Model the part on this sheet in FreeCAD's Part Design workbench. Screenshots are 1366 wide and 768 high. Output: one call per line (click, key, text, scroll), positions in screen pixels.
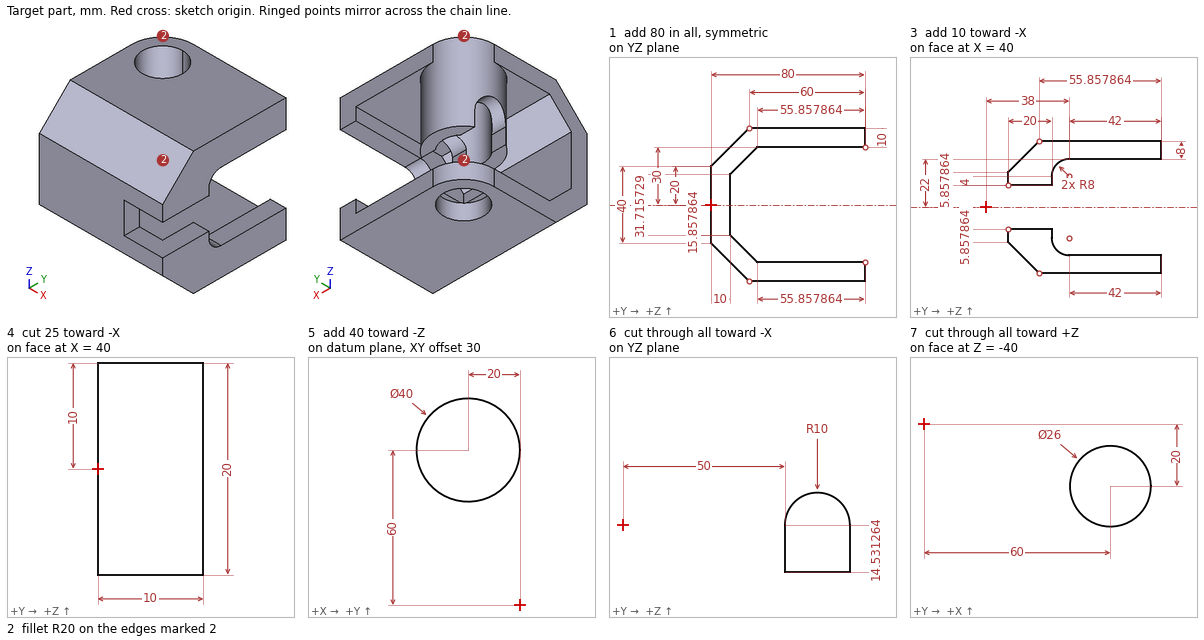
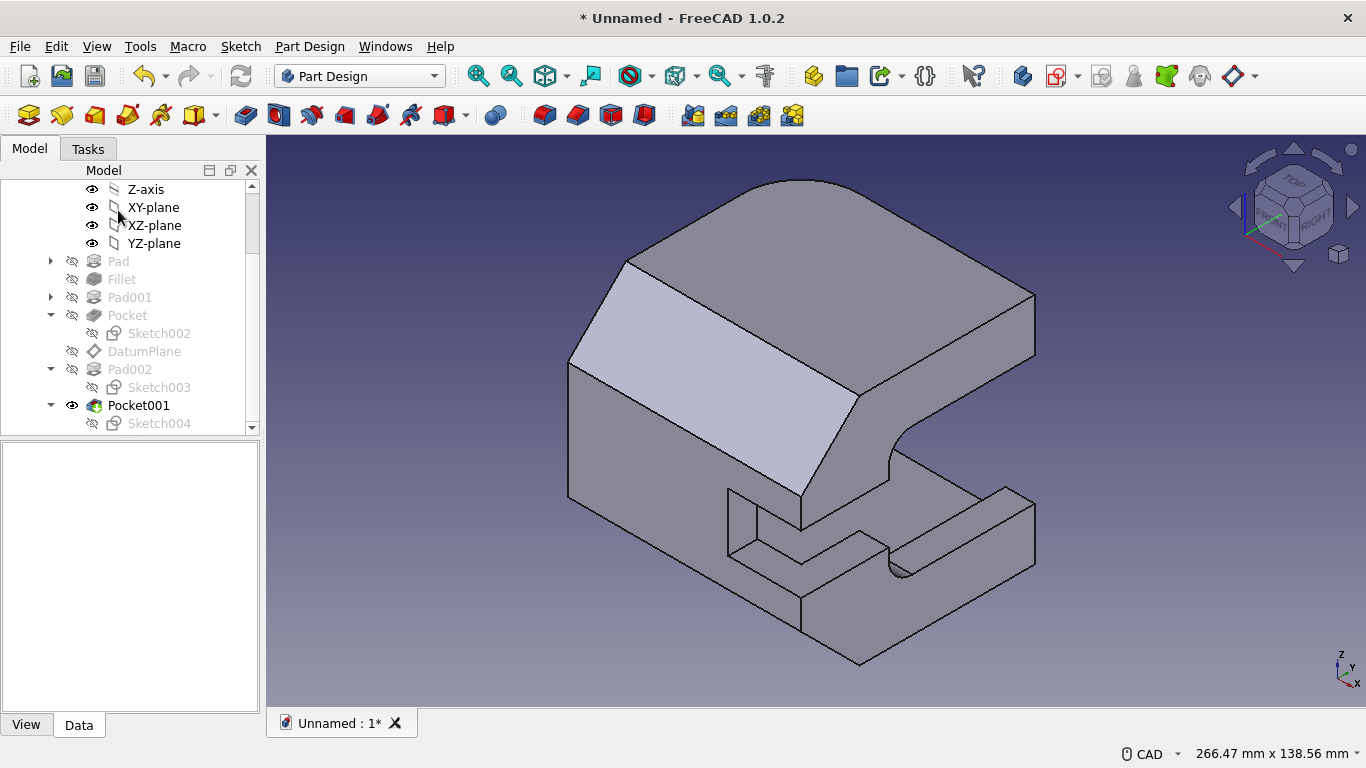
key(5)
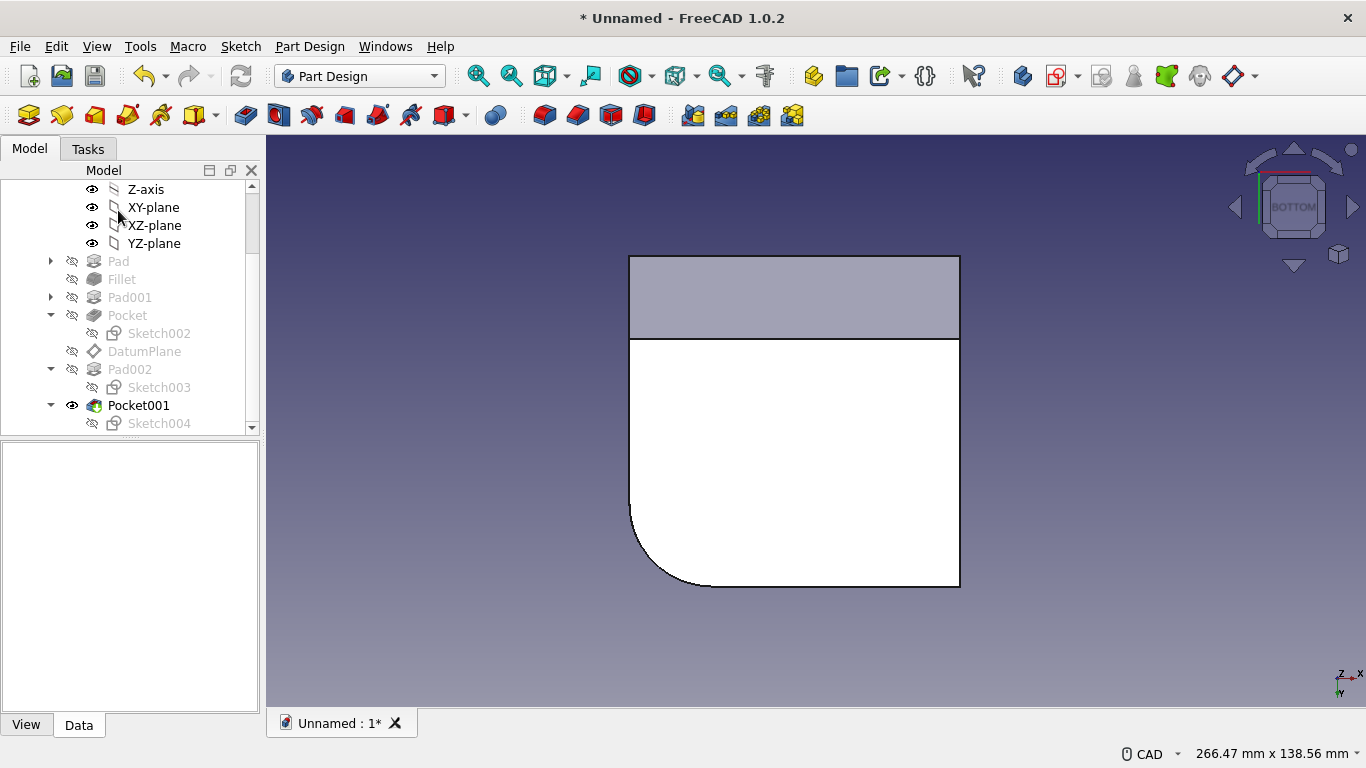
click(795, 462)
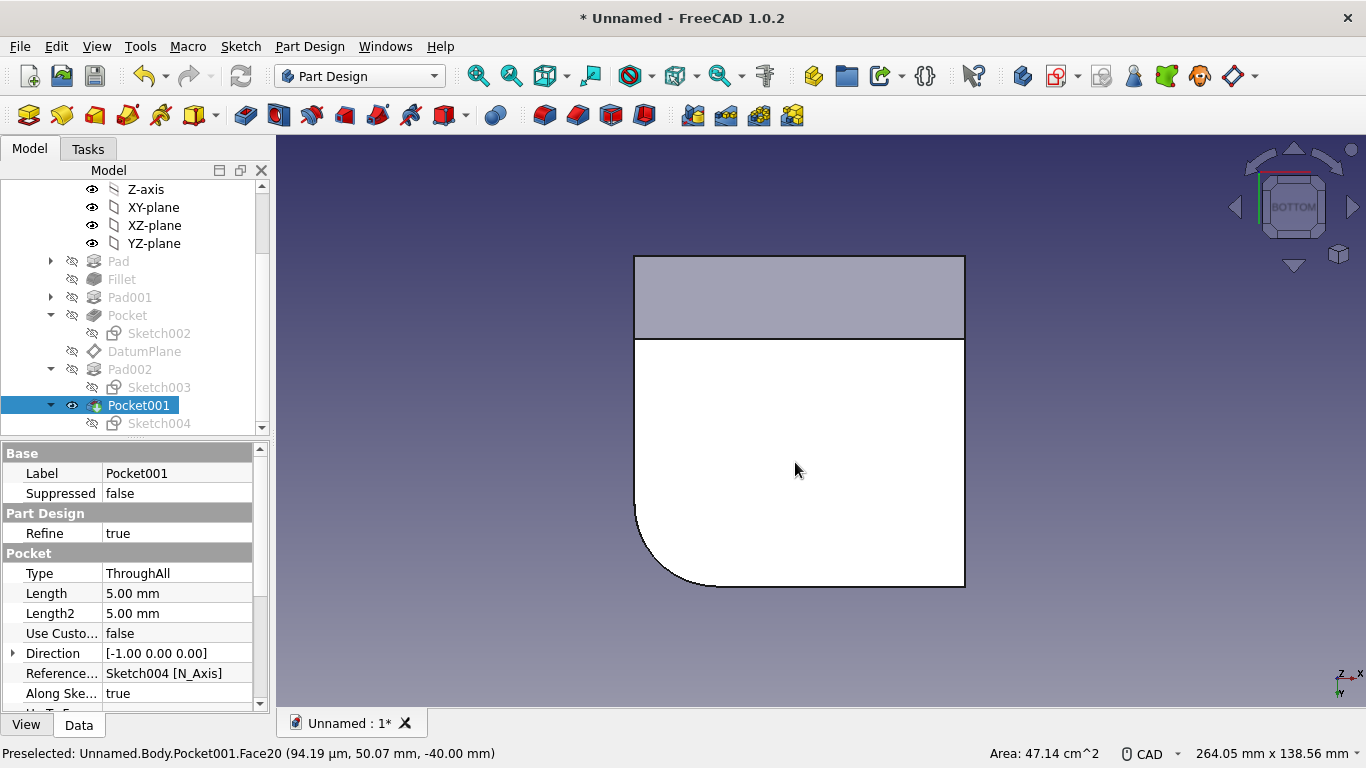
click(1056, 76)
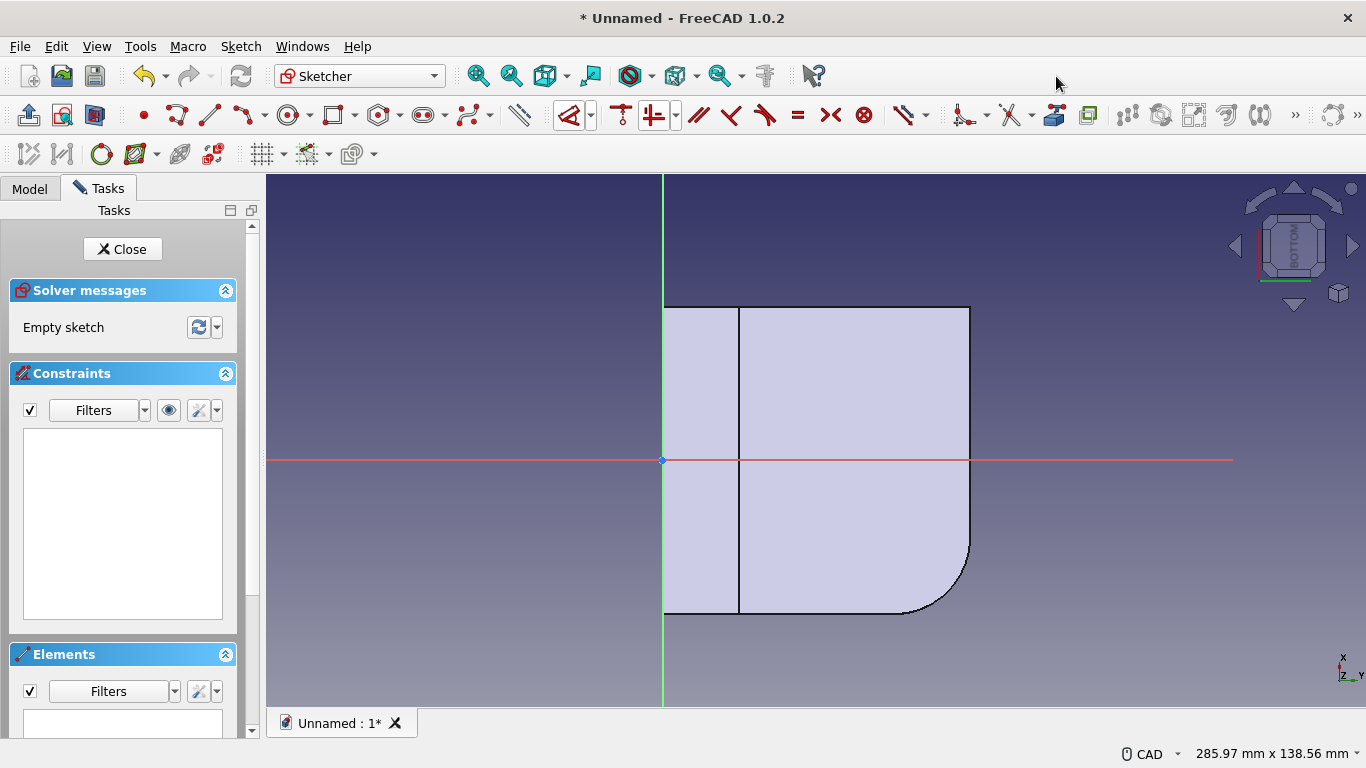
scroll(956, 579, up, 6)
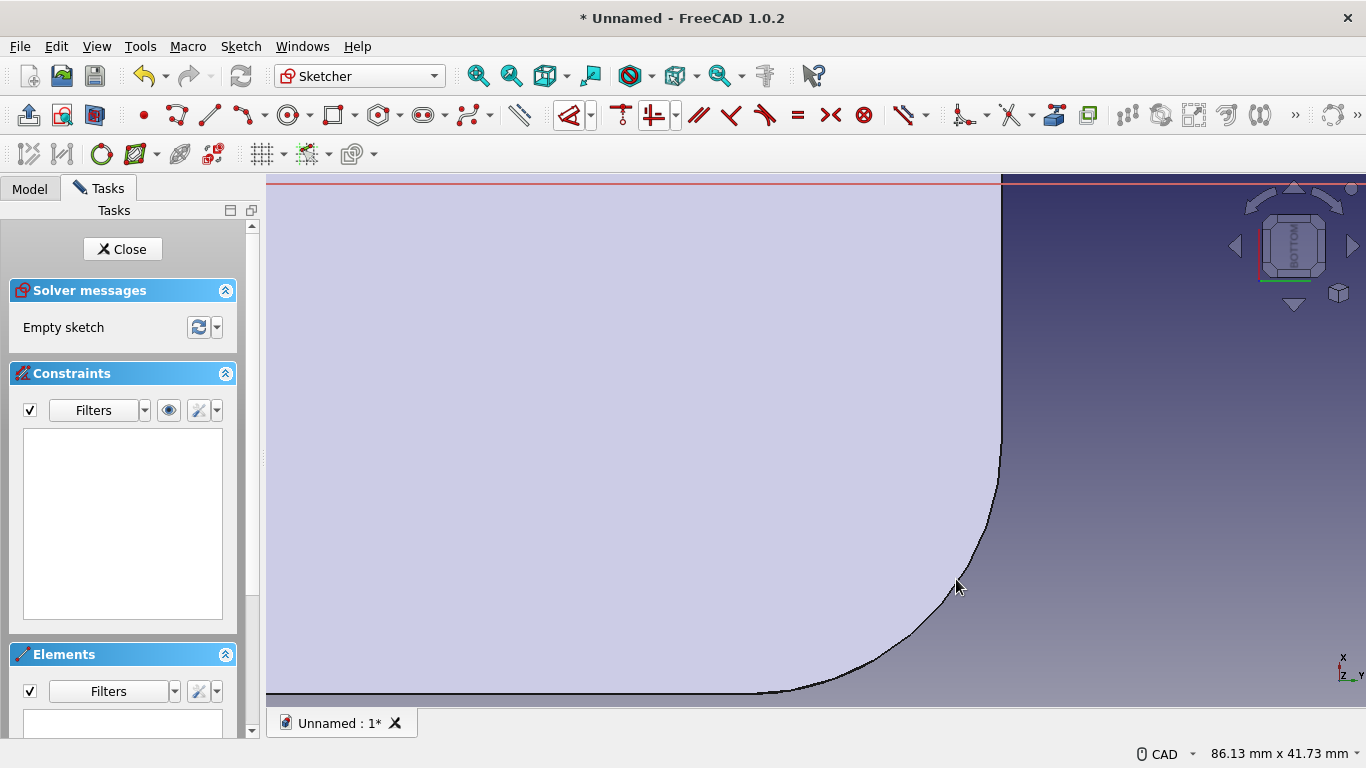
key(g)
key(c)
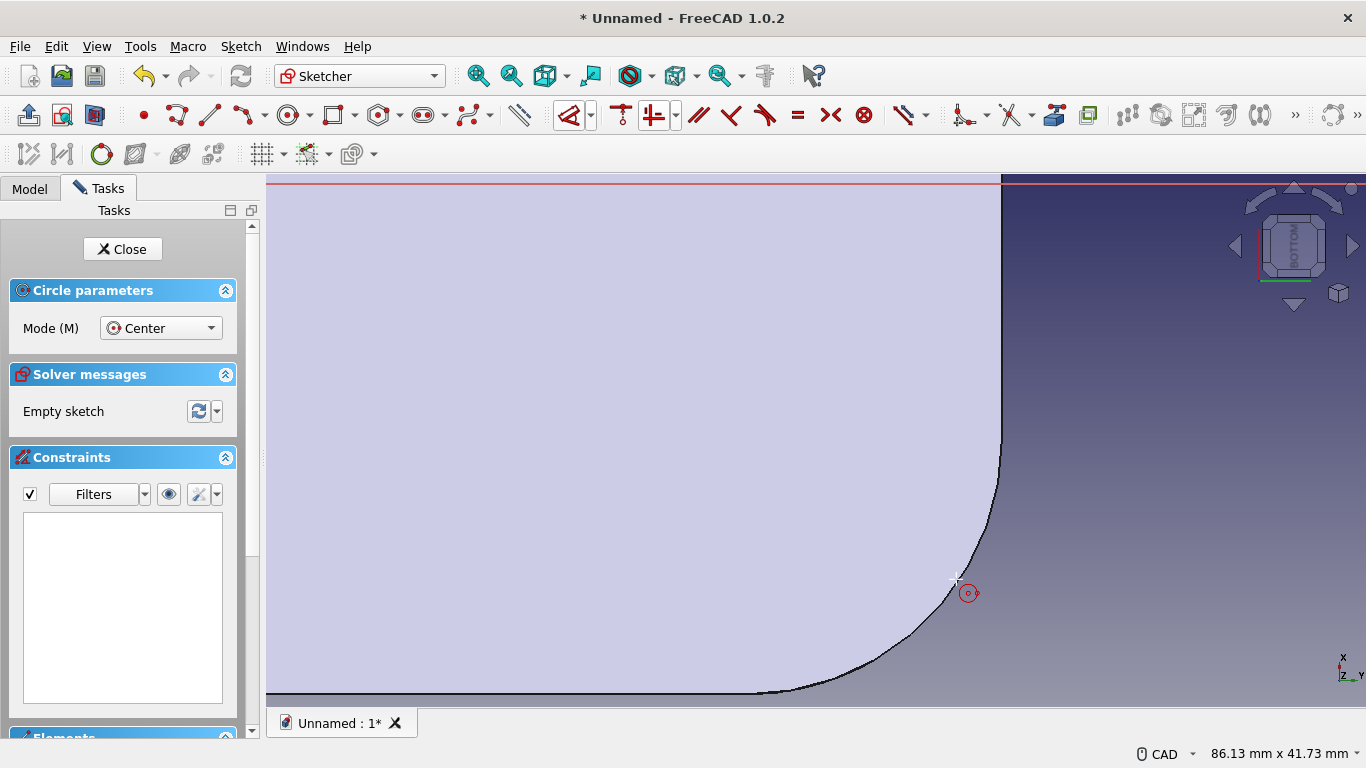
click(747, 439)
move(864, 322)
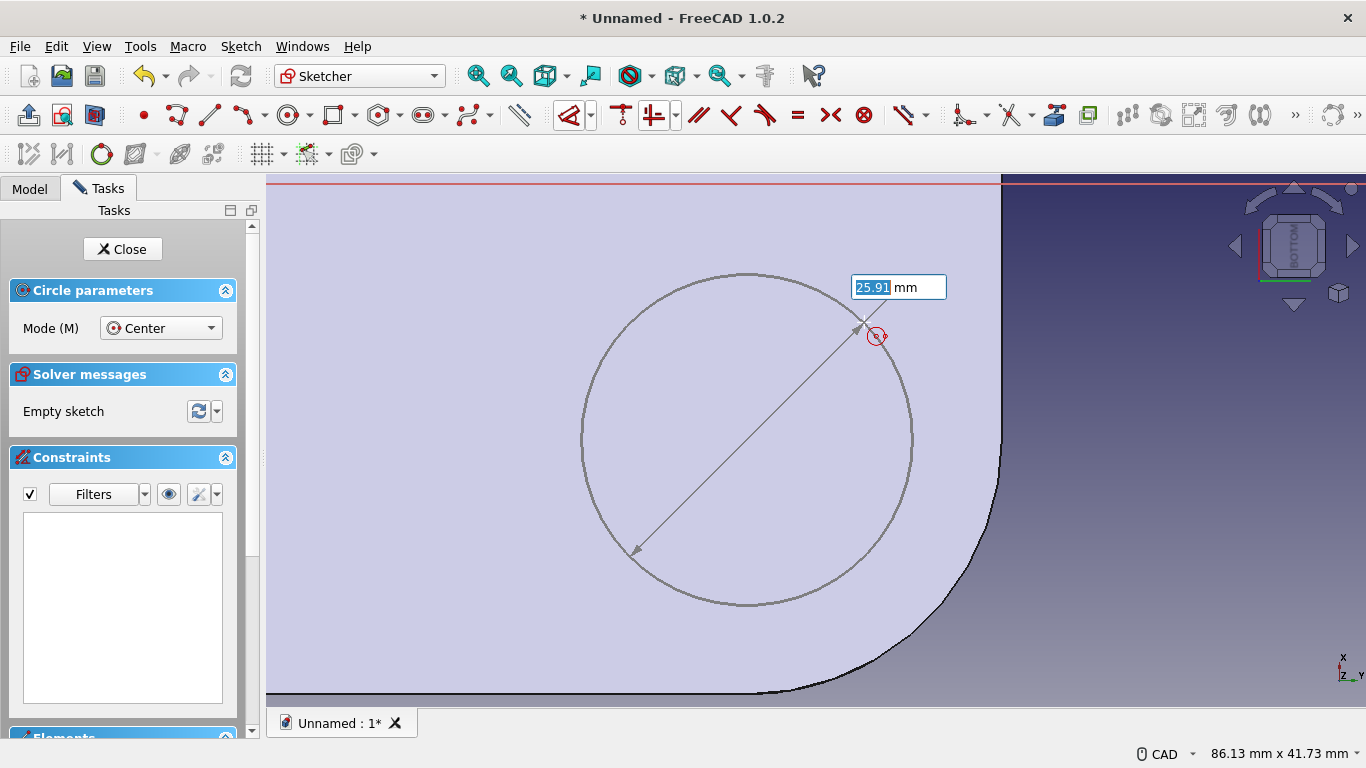
text(26)
key(Return)
key(Escape)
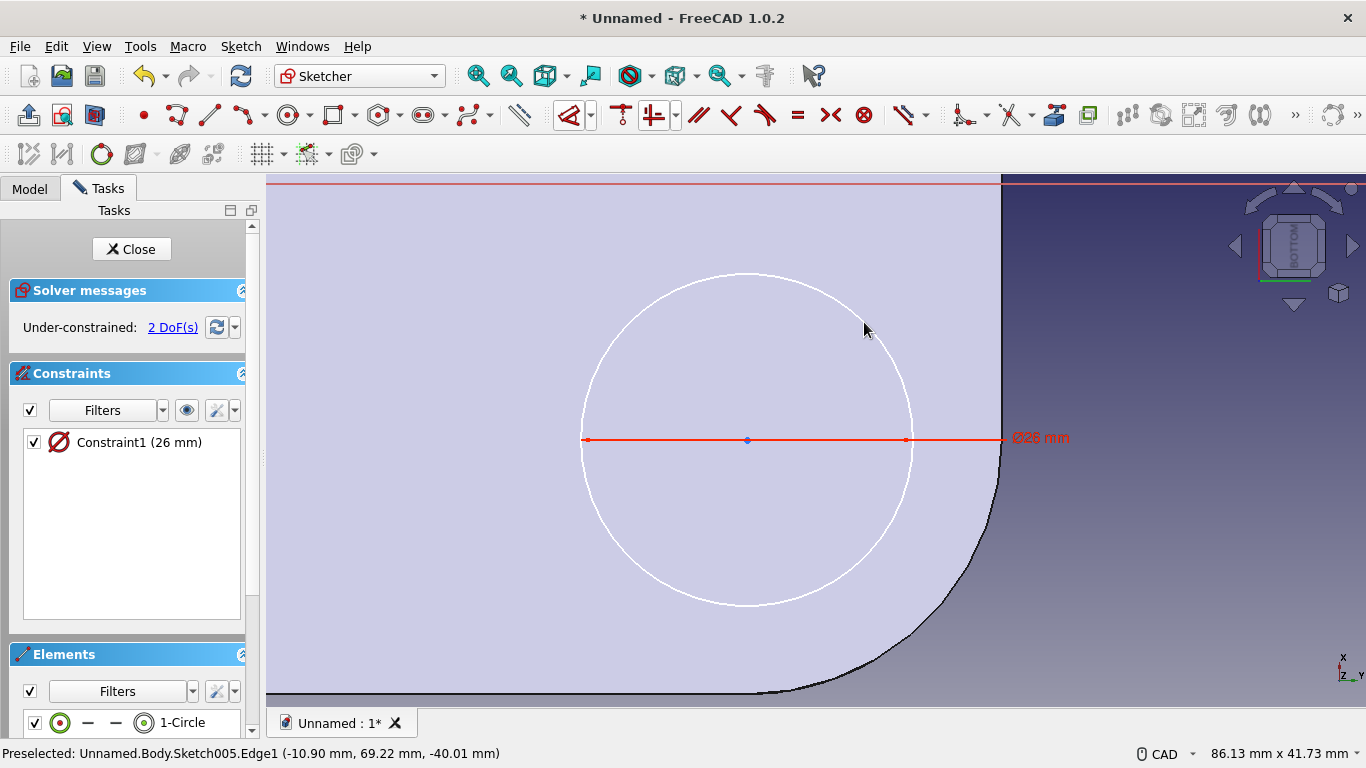
click(747, 440)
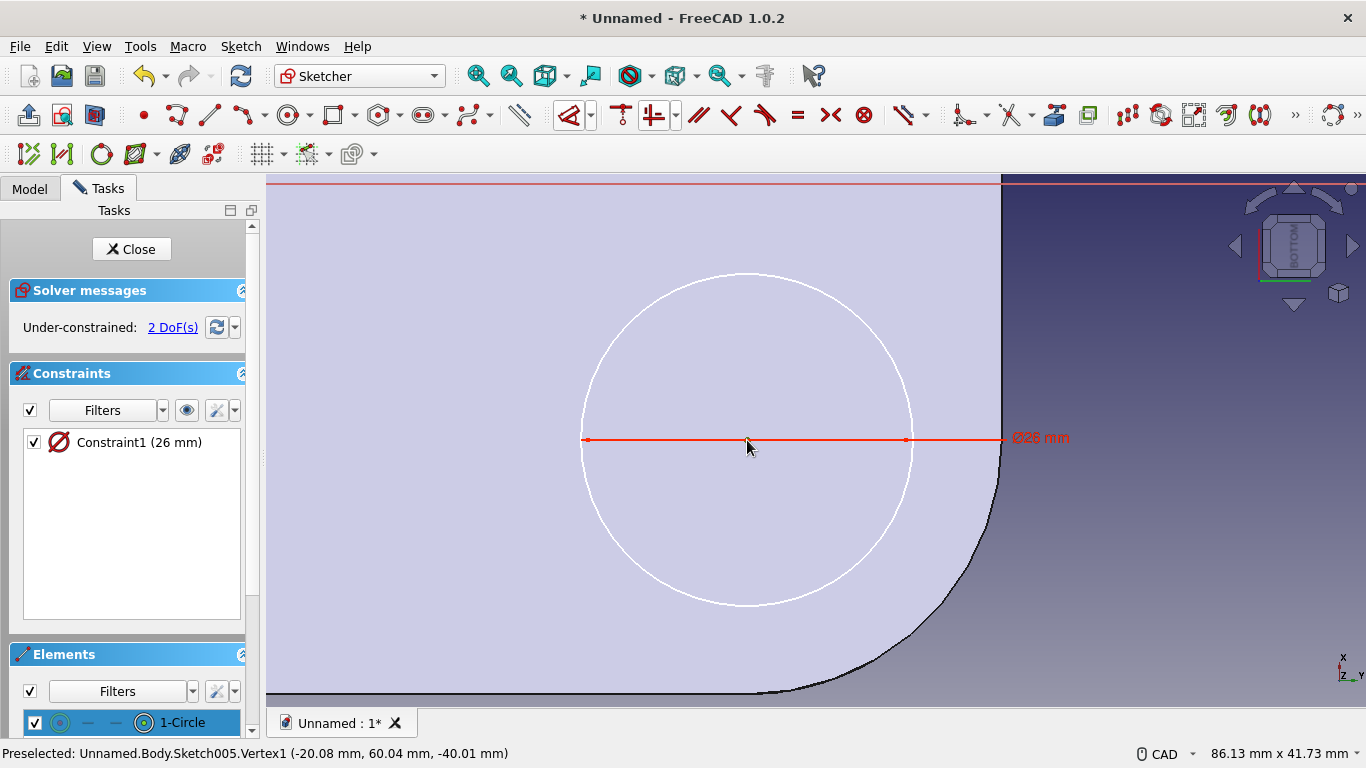
click(590, 116)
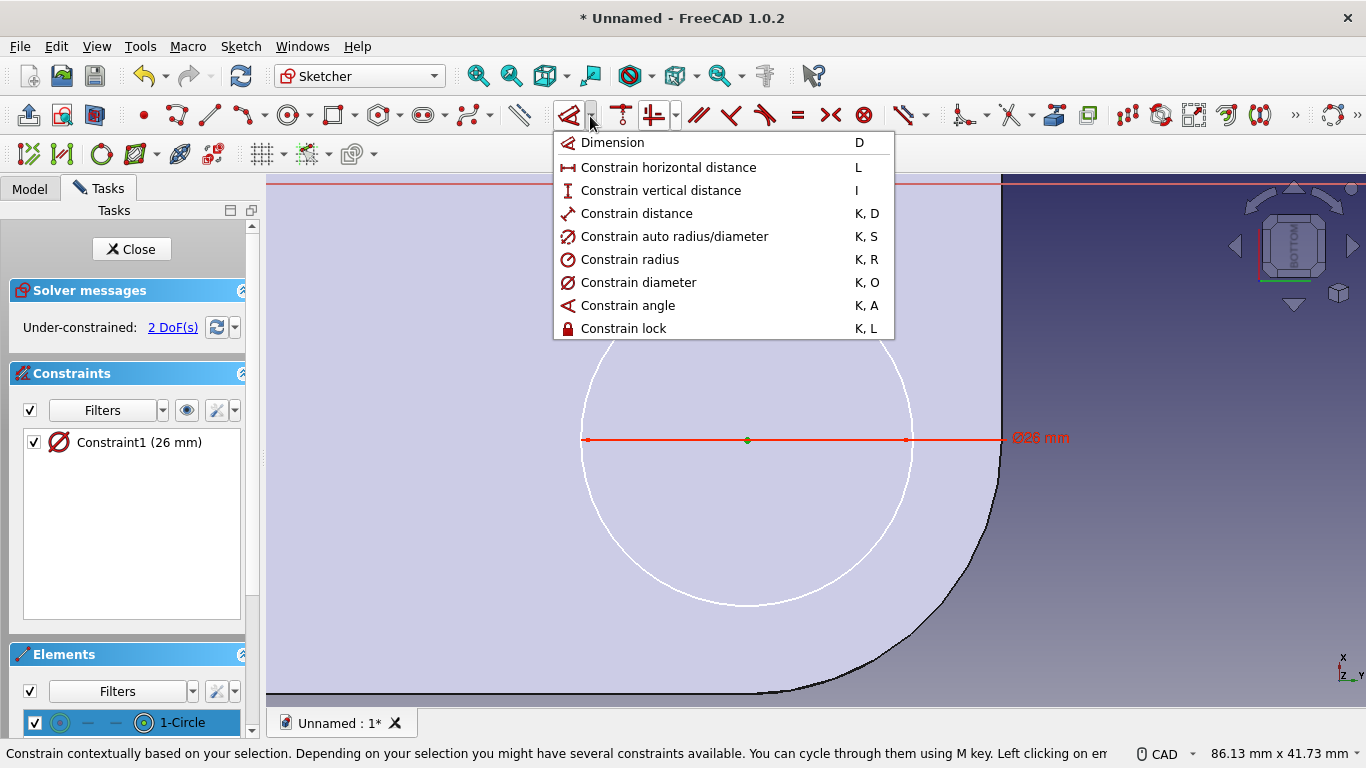
click(724, 168)